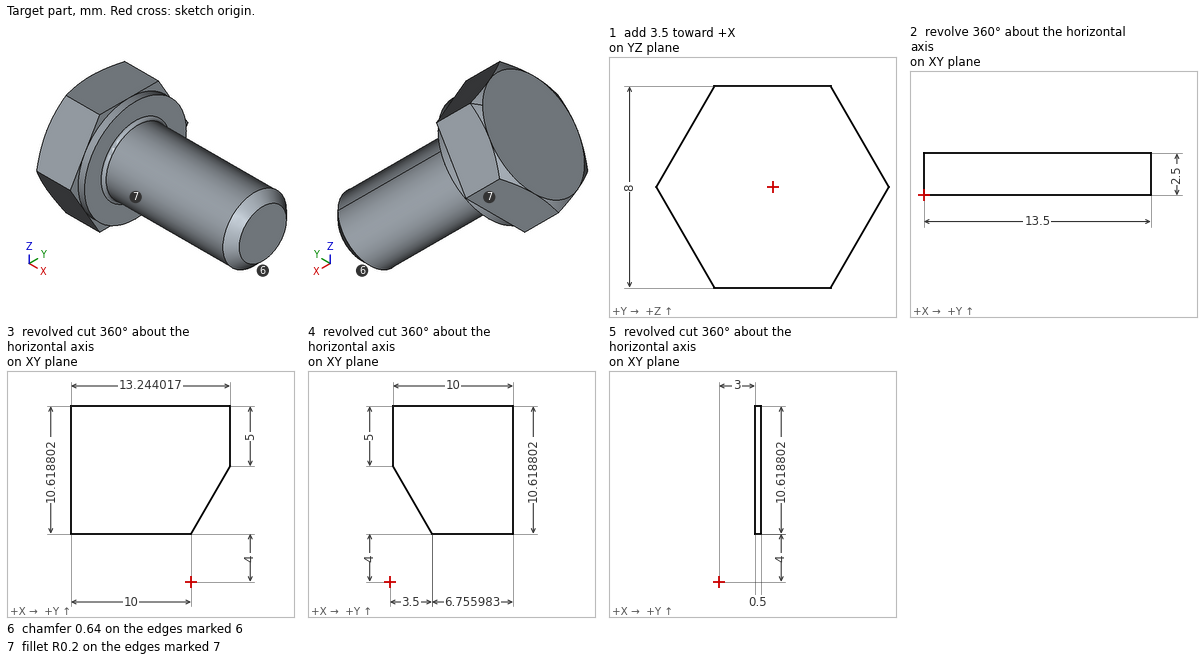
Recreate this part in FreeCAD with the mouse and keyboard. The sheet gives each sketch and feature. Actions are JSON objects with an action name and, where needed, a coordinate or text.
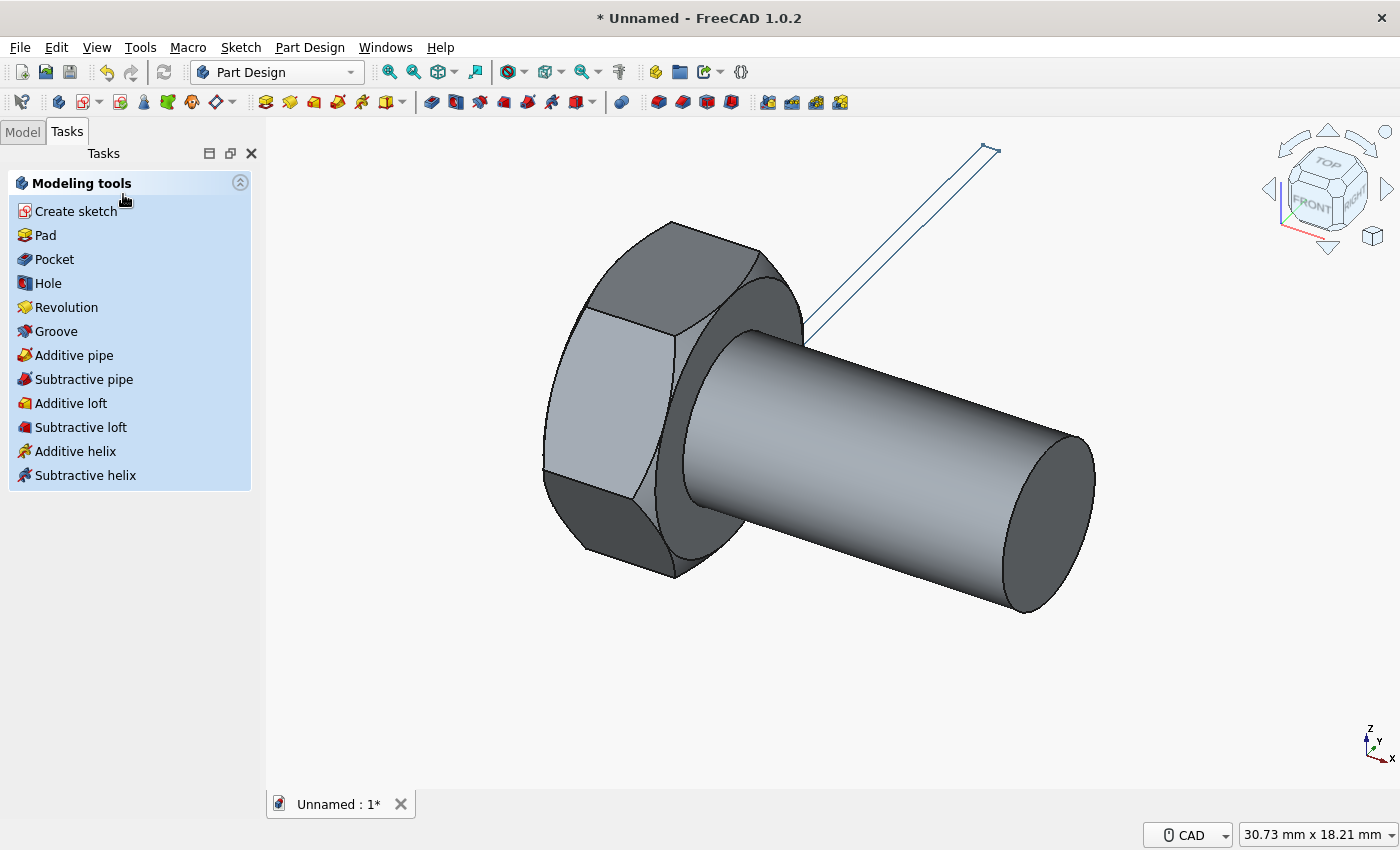
{"action": "left_click", "coordinate": [480, 102]}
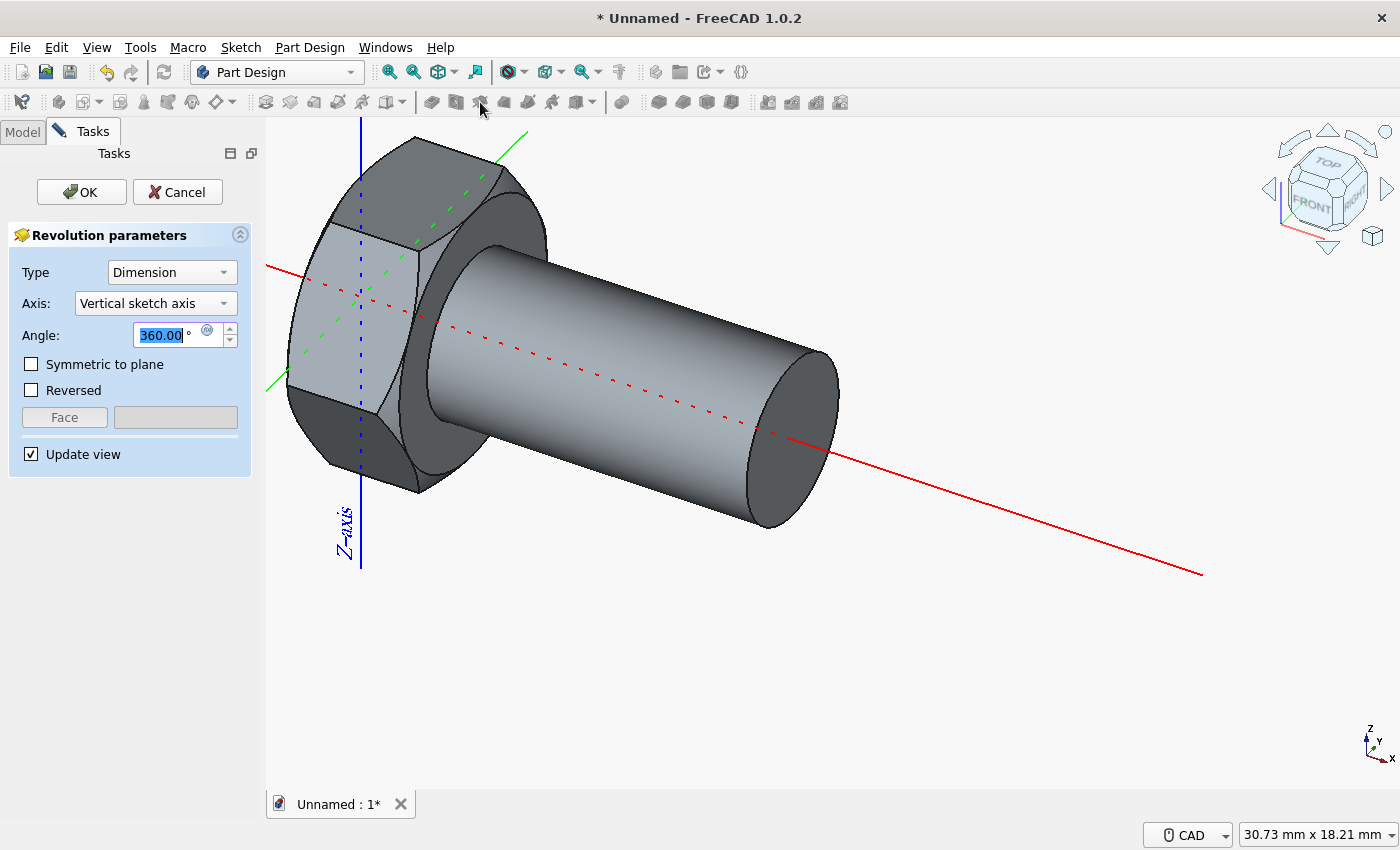
{"action": "left_click", "coordinate": [156, 304]}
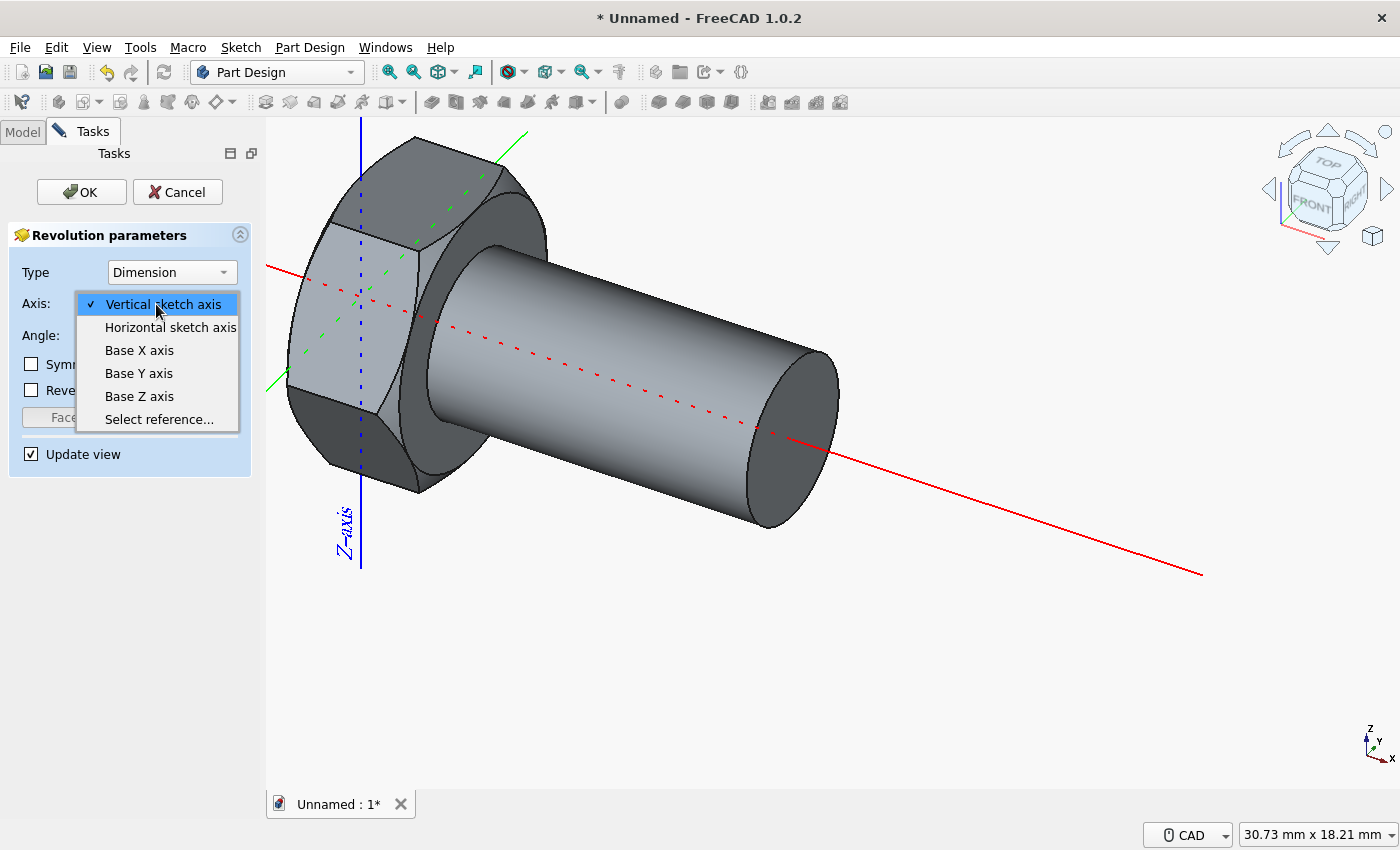
{"action": "left_click", "coordinate": [156, 328]}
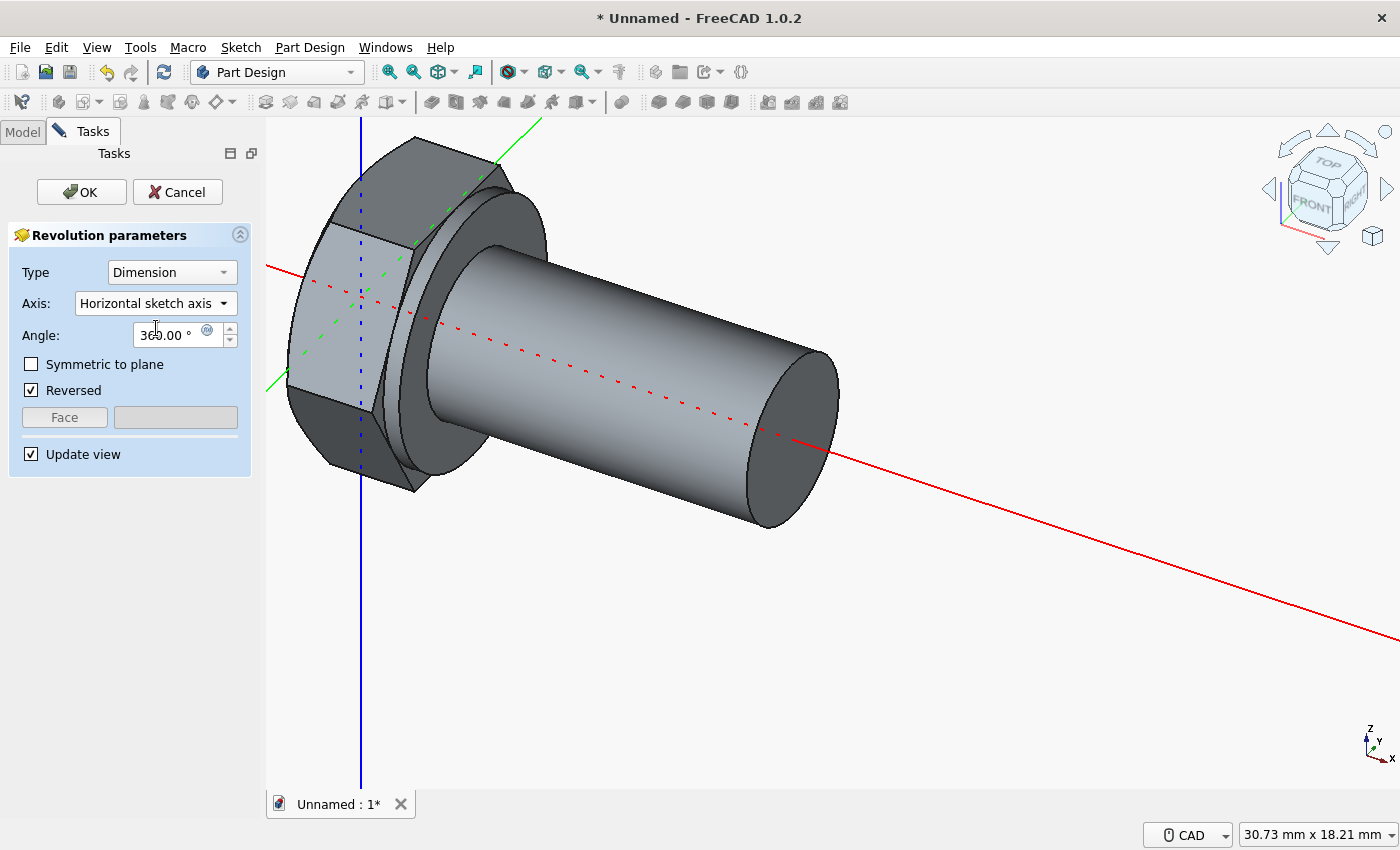
{"action": "left_click", "coordinate": [82, 192]}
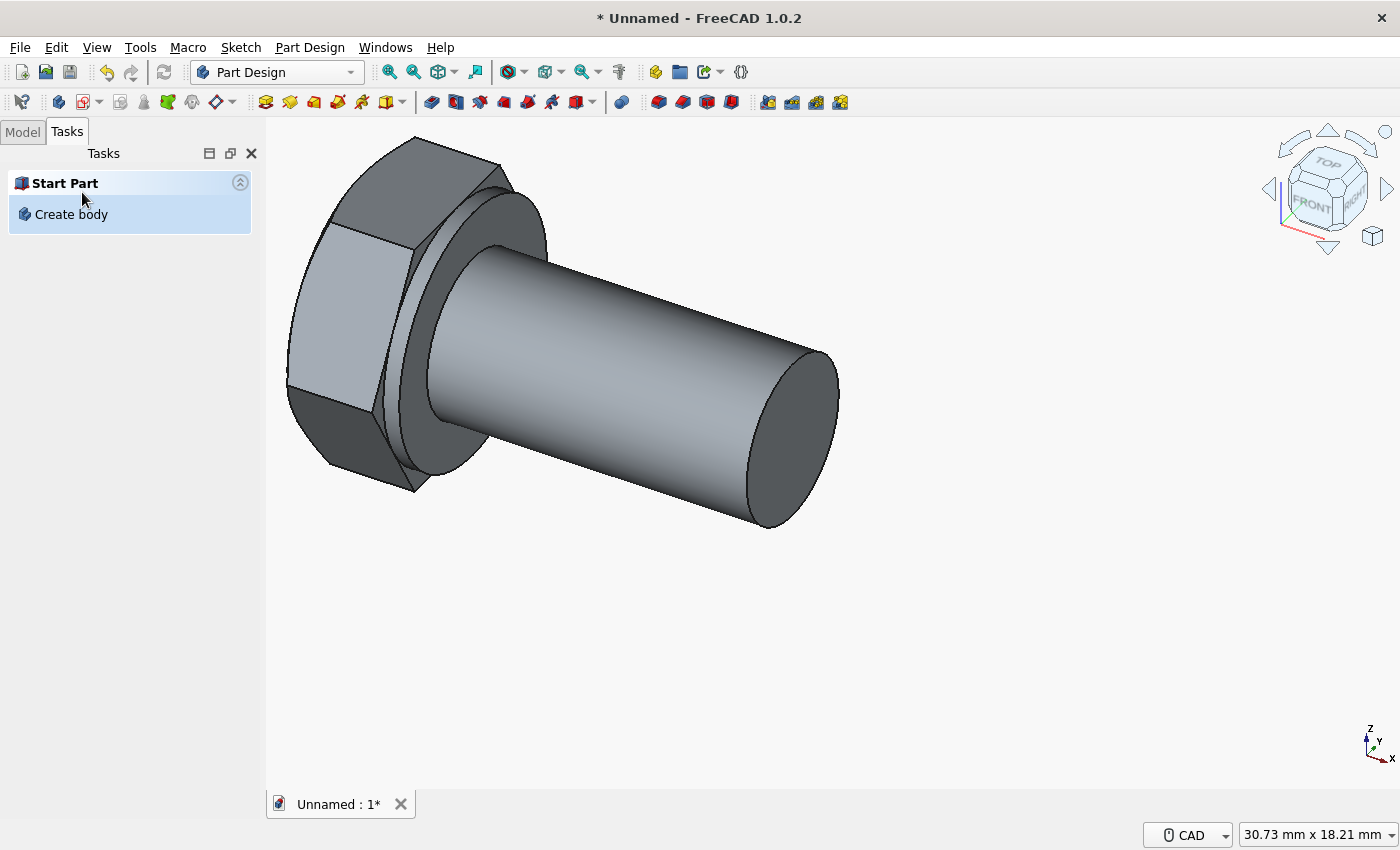
{"action": "left_click", "coordinate": [390, 72]}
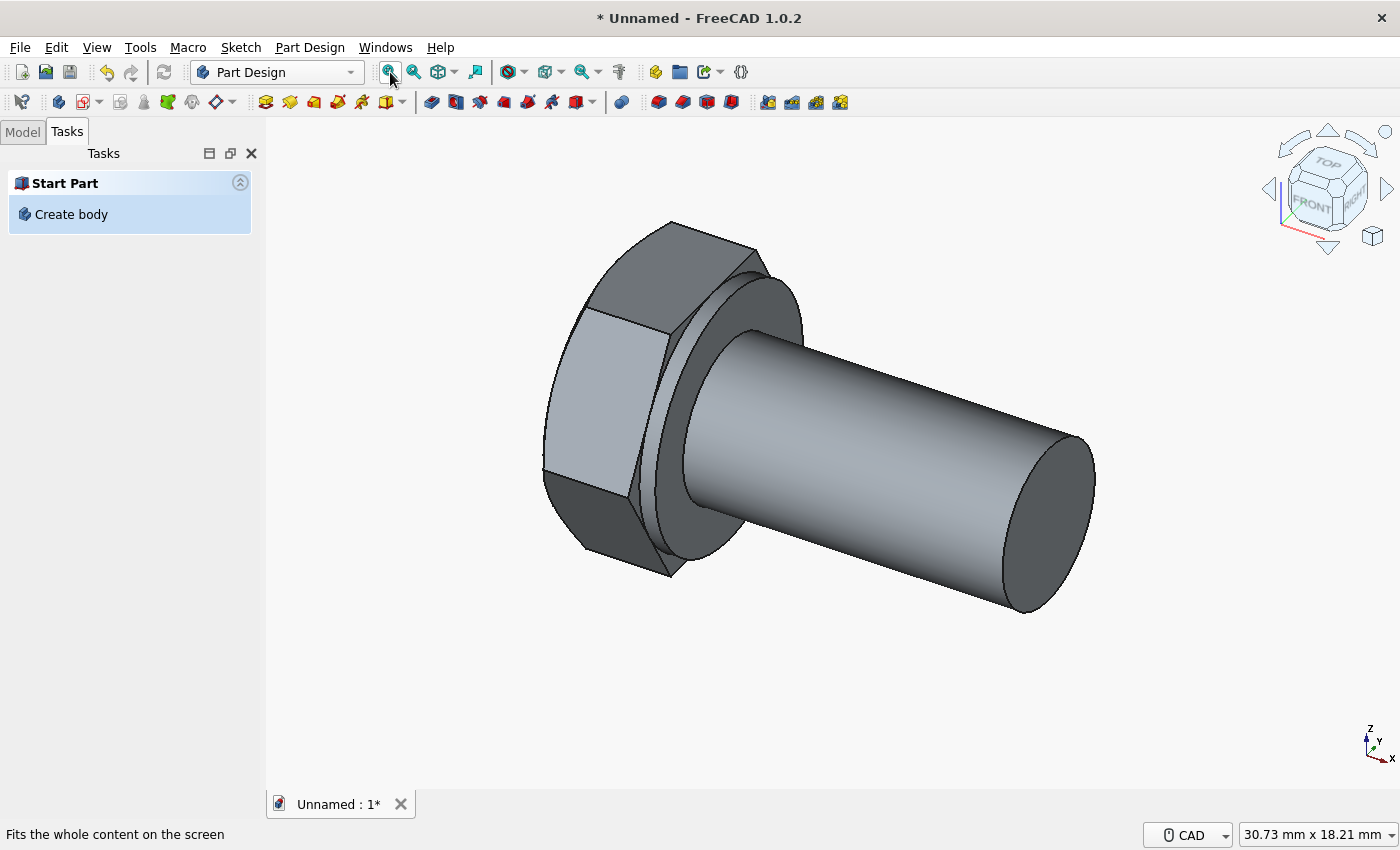
{"action": "left_click", "coordinate": [1003, 569]}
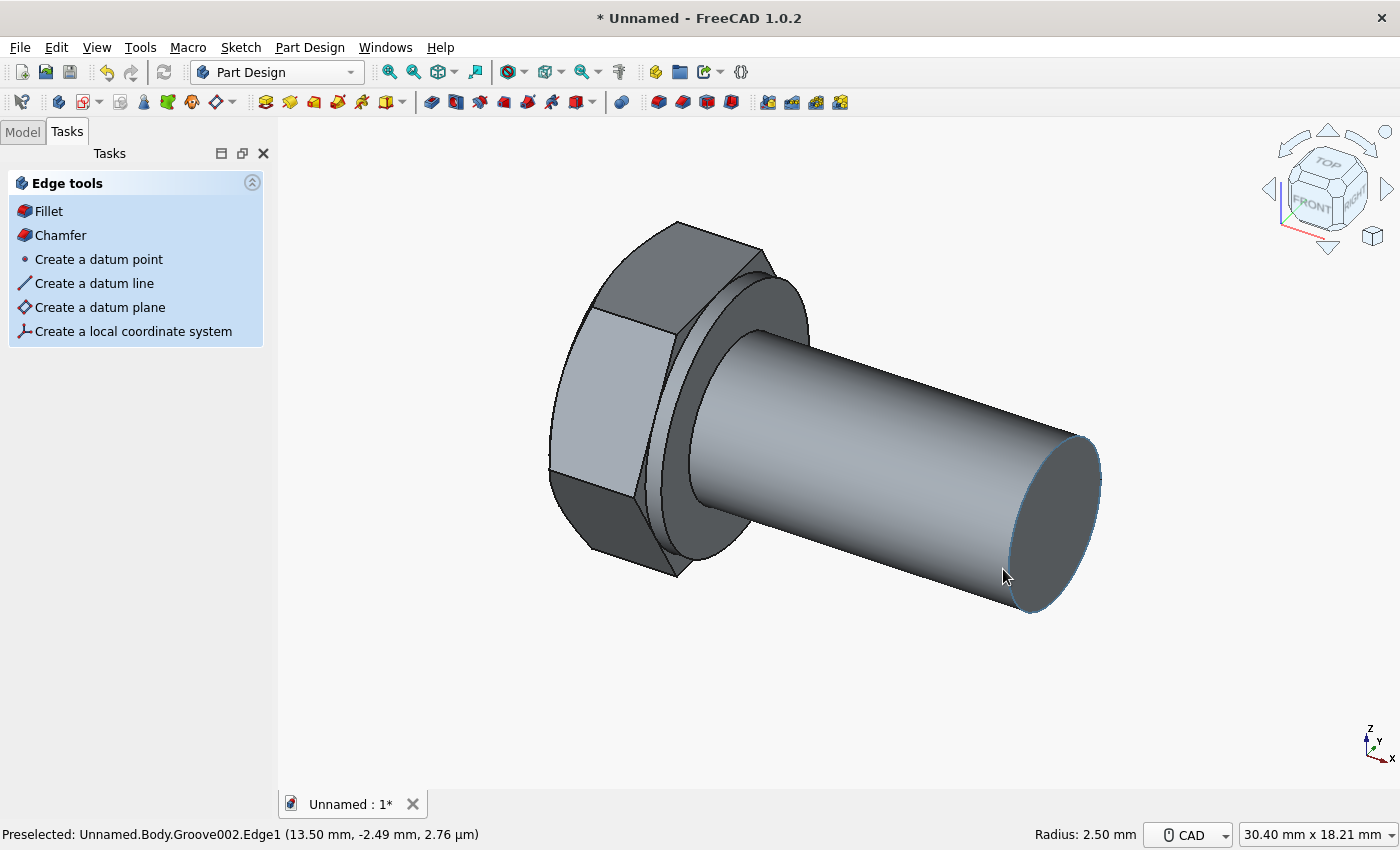
{"action": "left_click", "coordinate": [684, 102]}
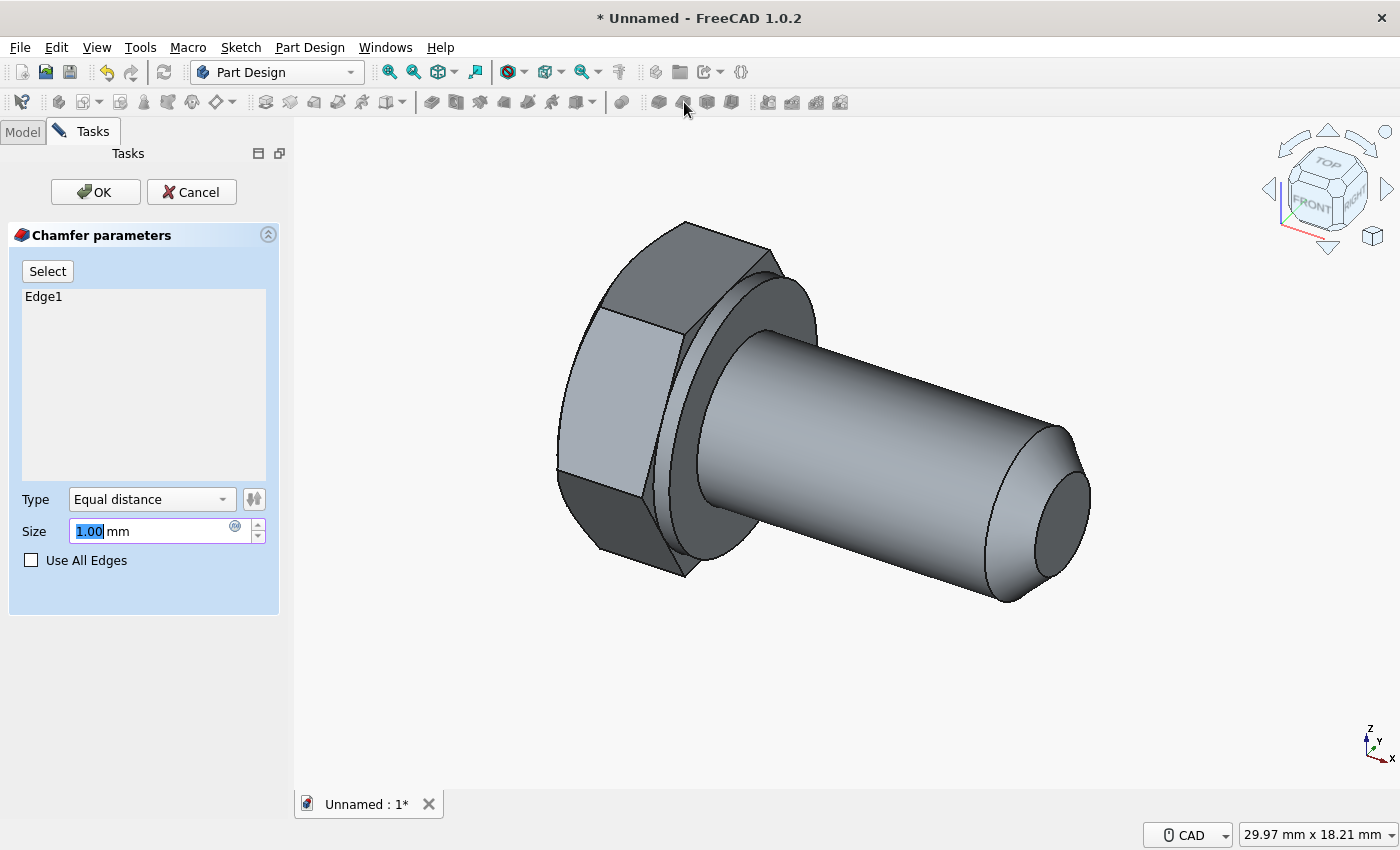
{"action": "type", "text": "0.64"}
{"action": "key", "text": "Tab"}